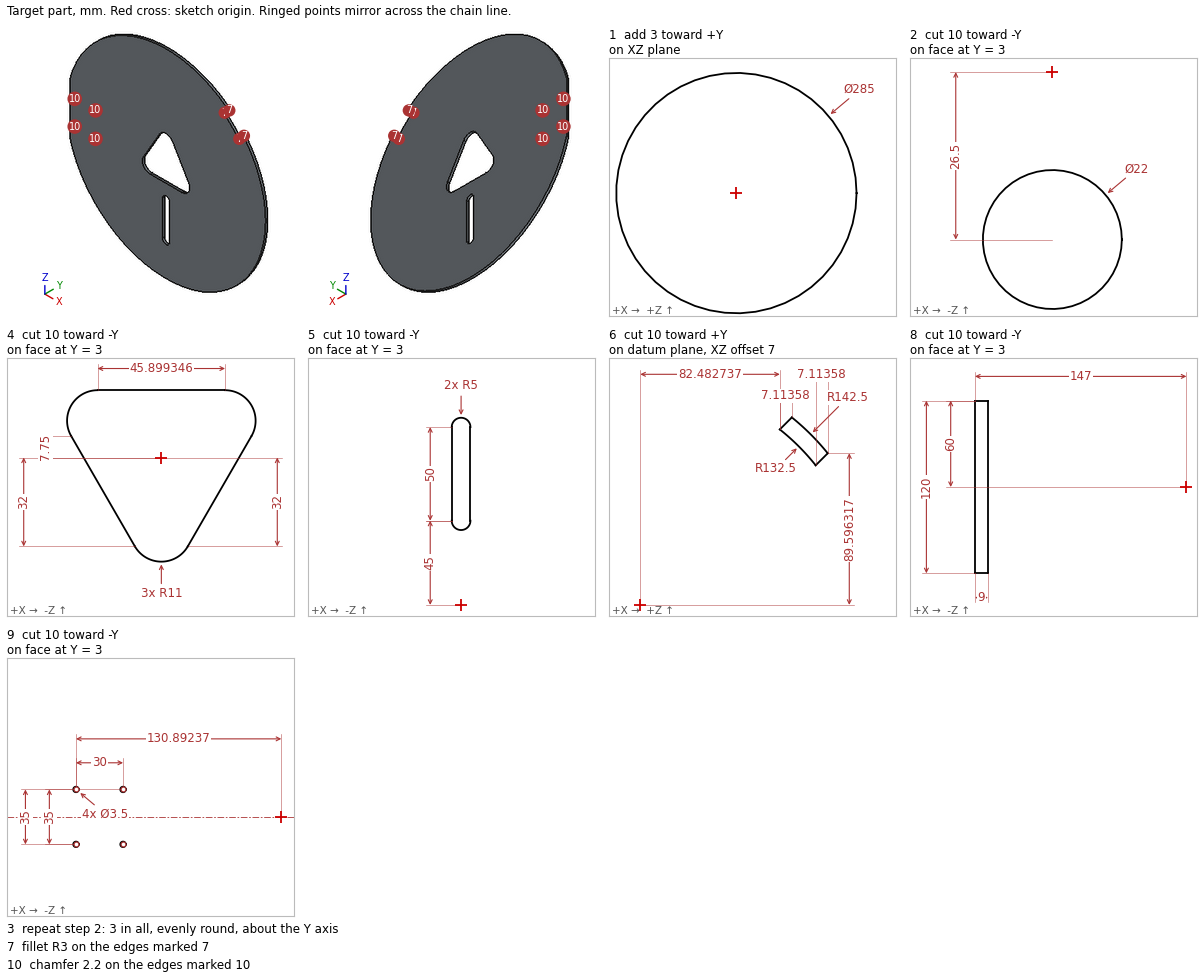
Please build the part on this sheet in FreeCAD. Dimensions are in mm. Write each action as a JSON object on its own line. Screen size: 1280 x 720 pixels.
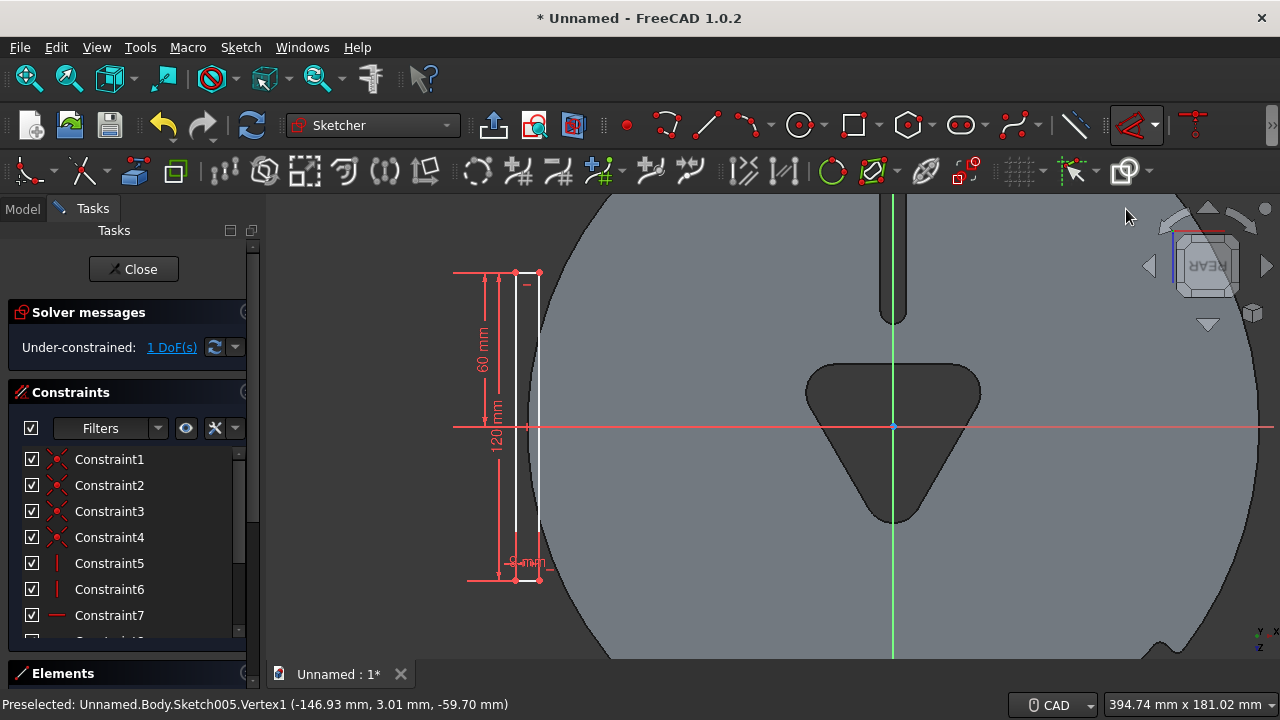
{"action": "left_click", "coordinate": [516, 273]}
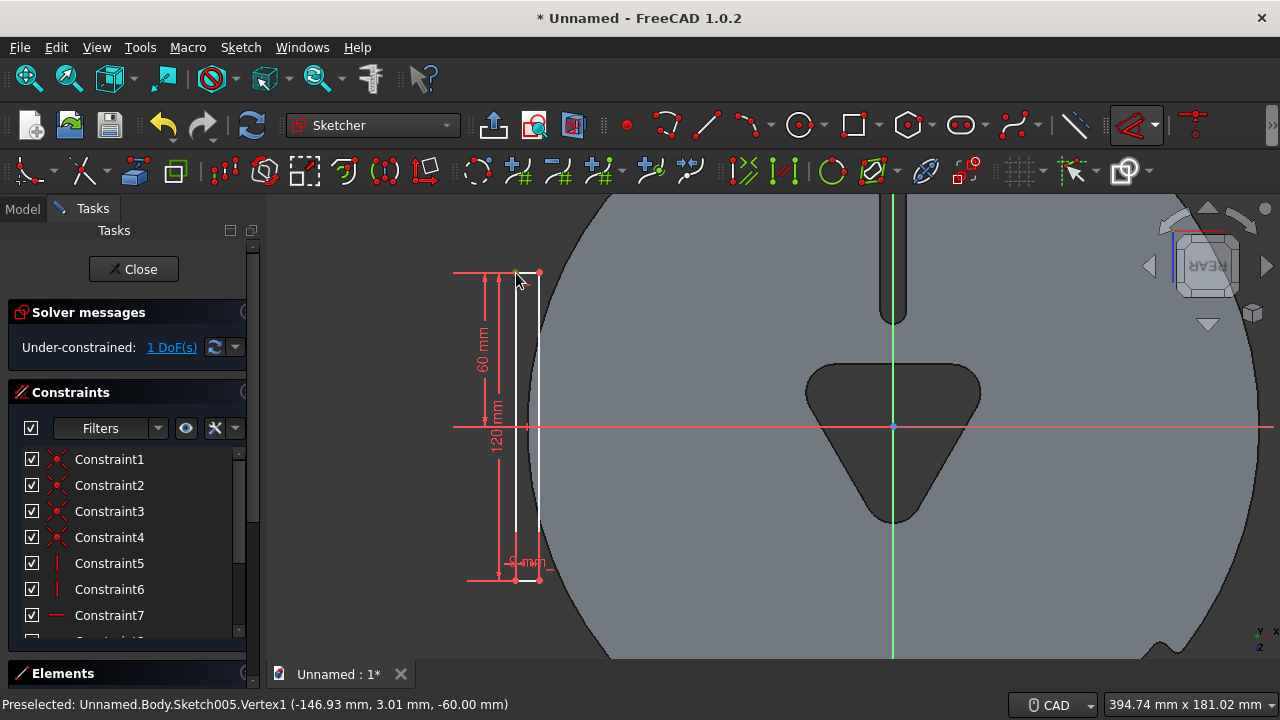
{"action": "left_click", "coordinate": [1158, 126]}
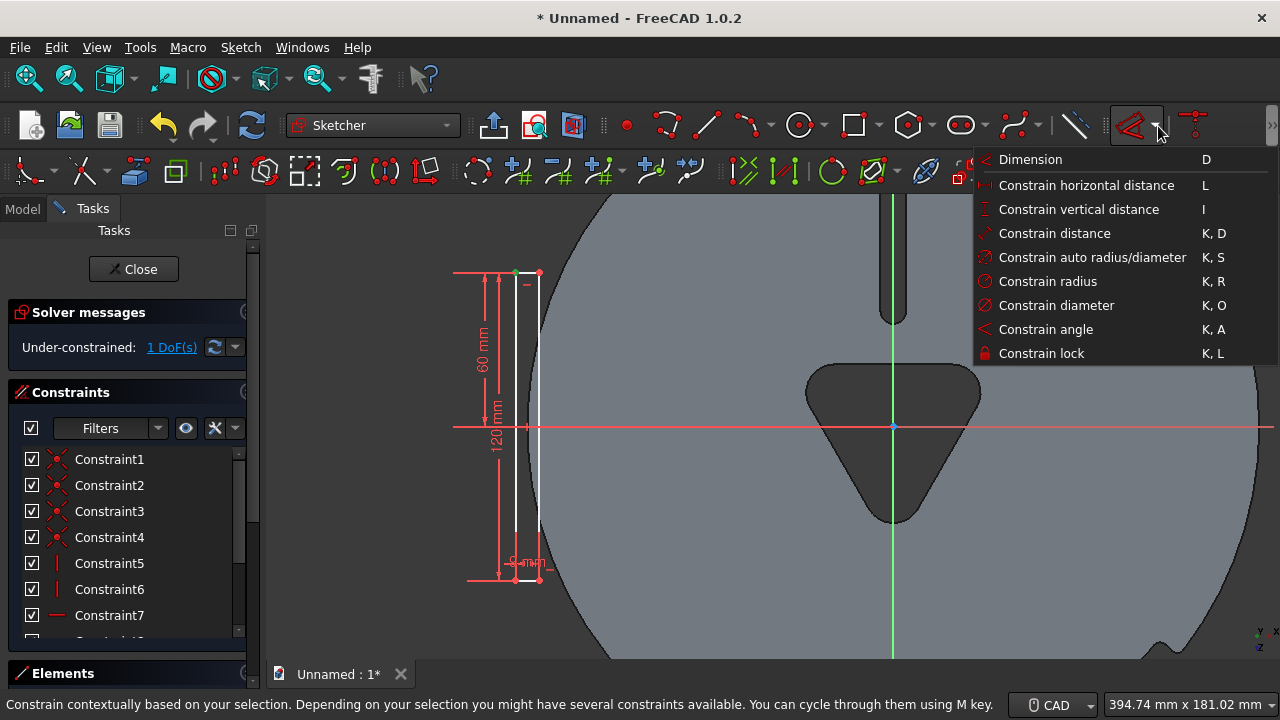
{"action": "left_click", "coordinate": [1126, 185]}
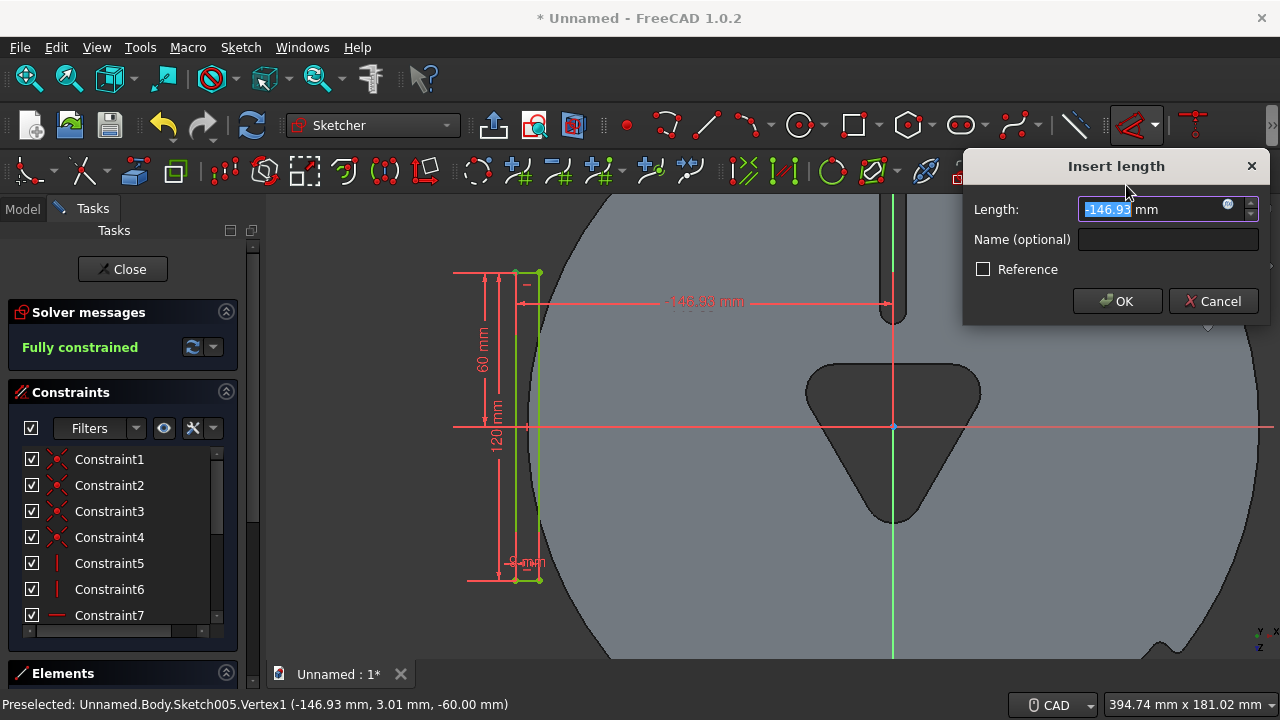
{"action": "type", "text": "-147"}
{"action": "key", "text": "Return"}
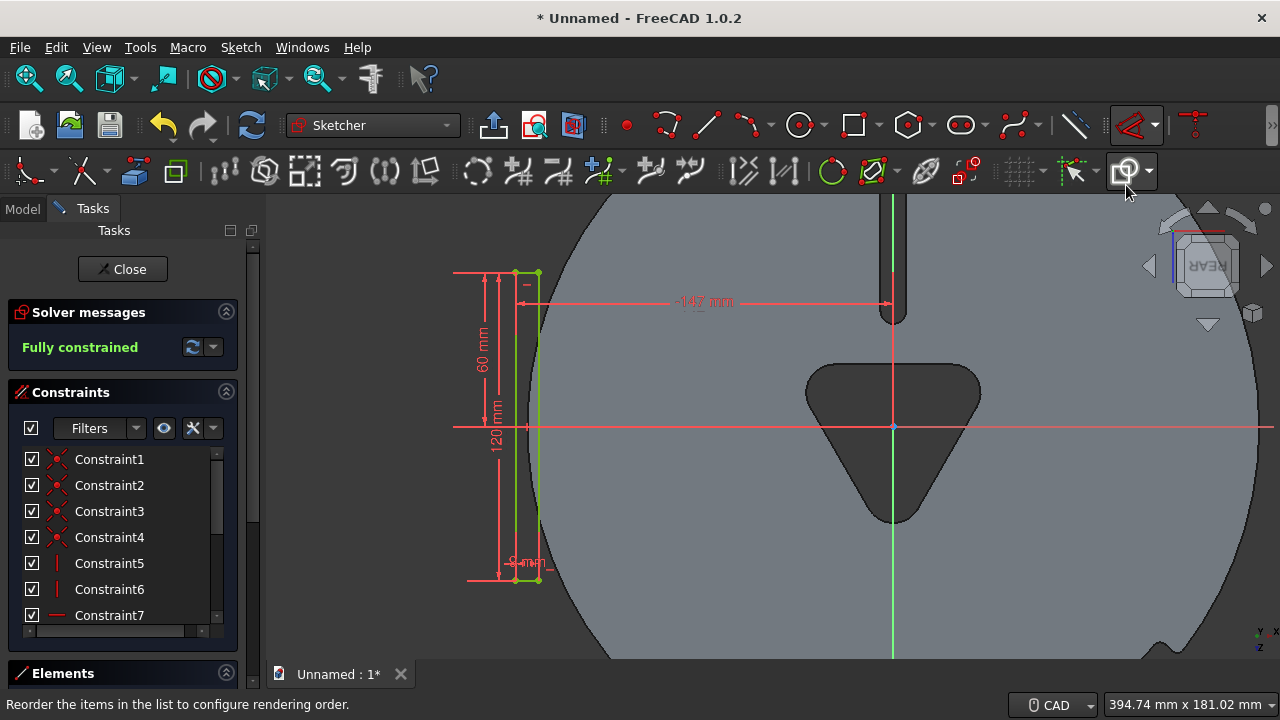
{"action": "left_click", "coordinate": [123, 269]}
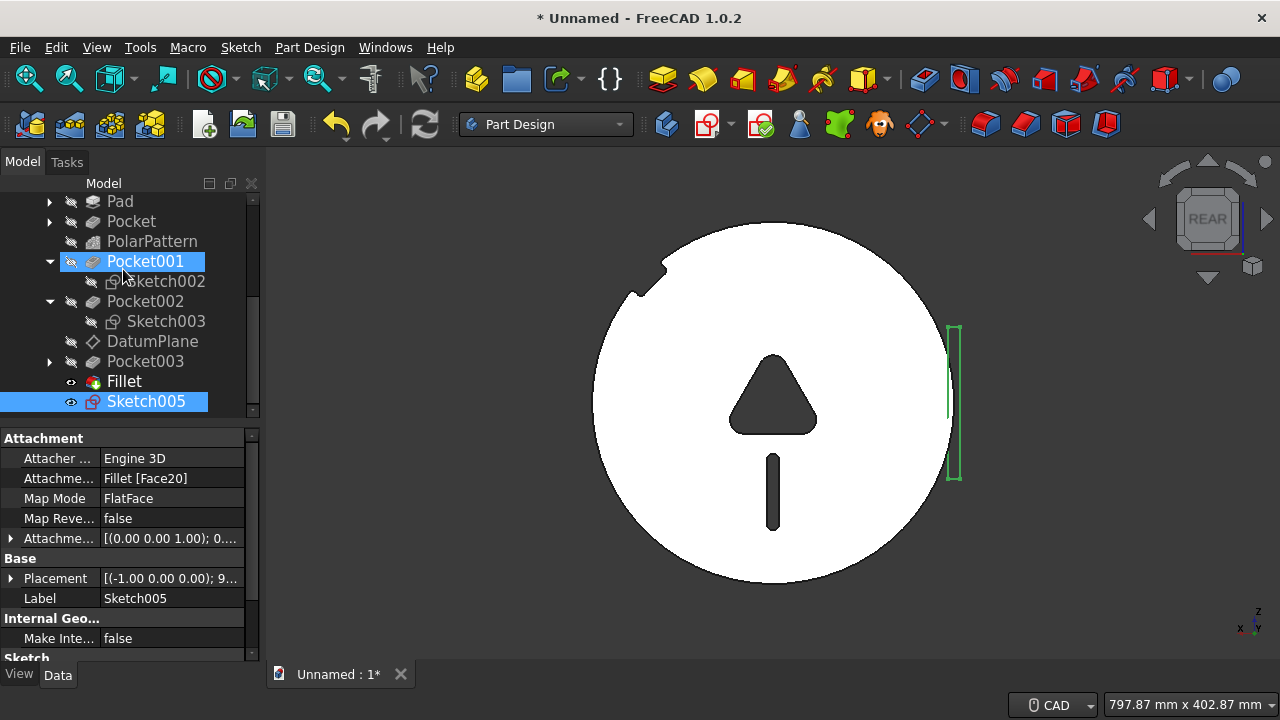
{"action": "left_click", "coordinate": [926, 80]}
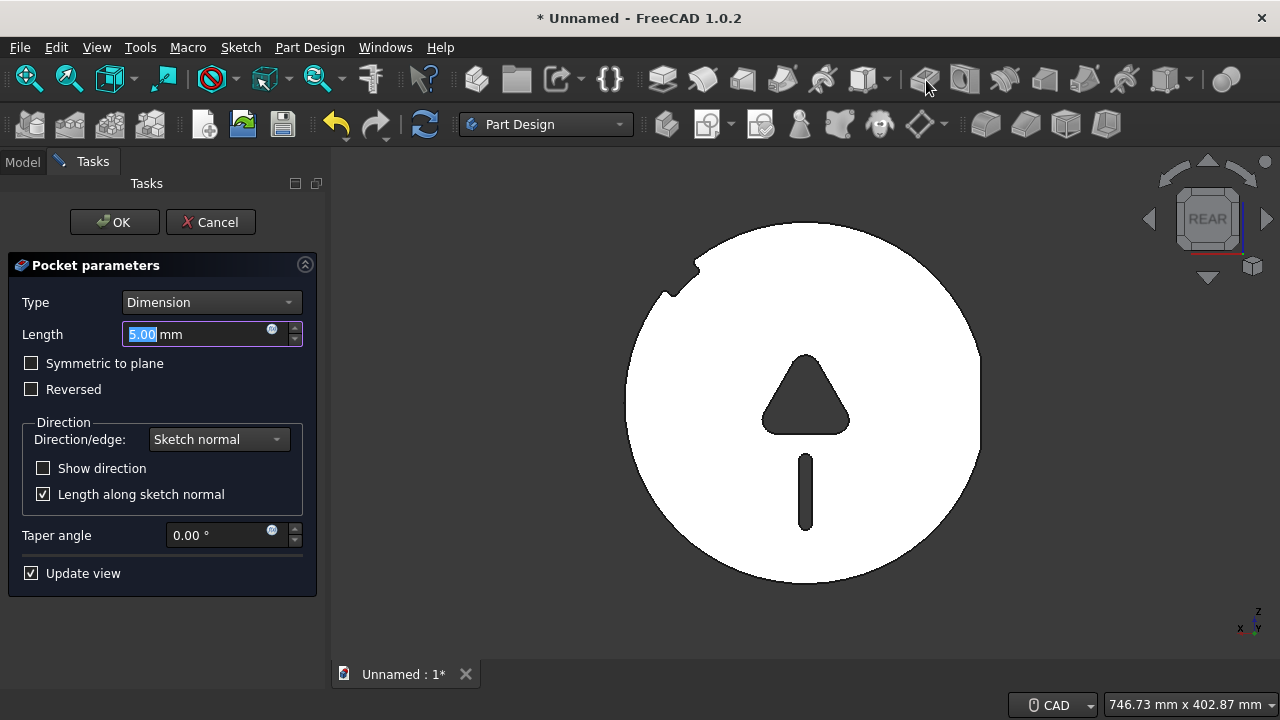
{"action": "type", "text": "10"}
{"action": "key", "text": "Tab"}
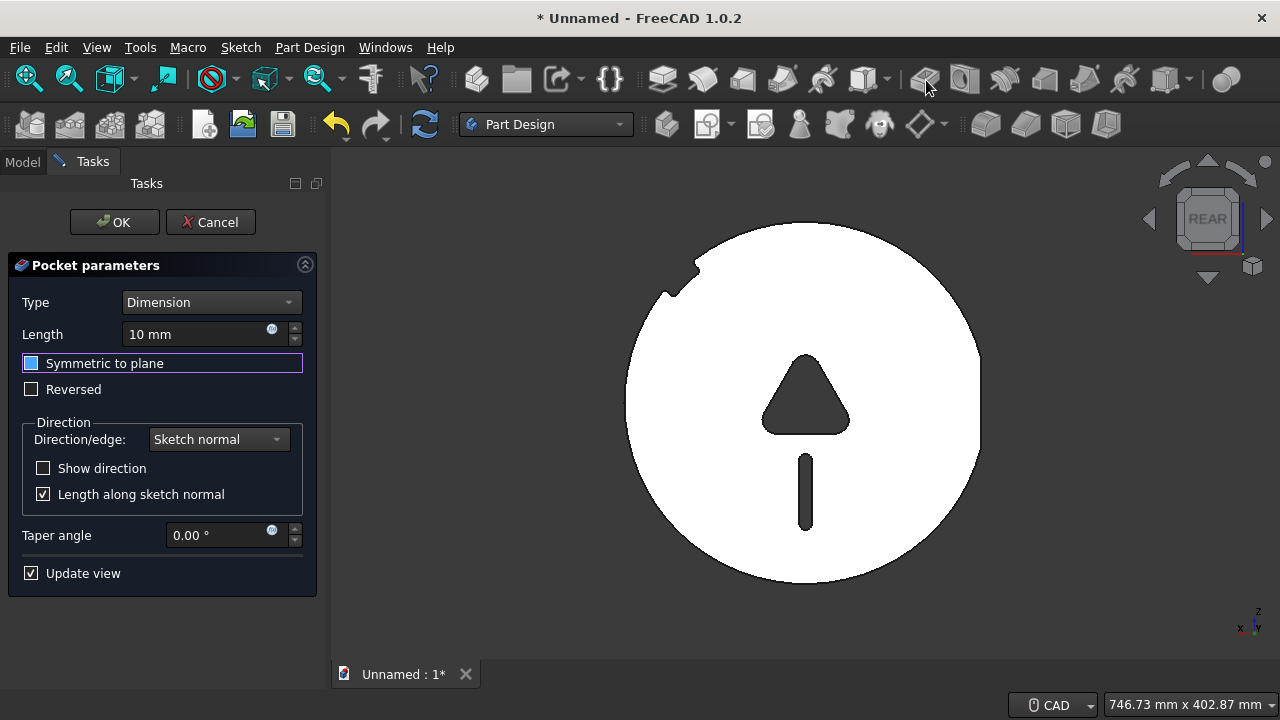
{"action": "left_click", "coordinate": [115, 222]}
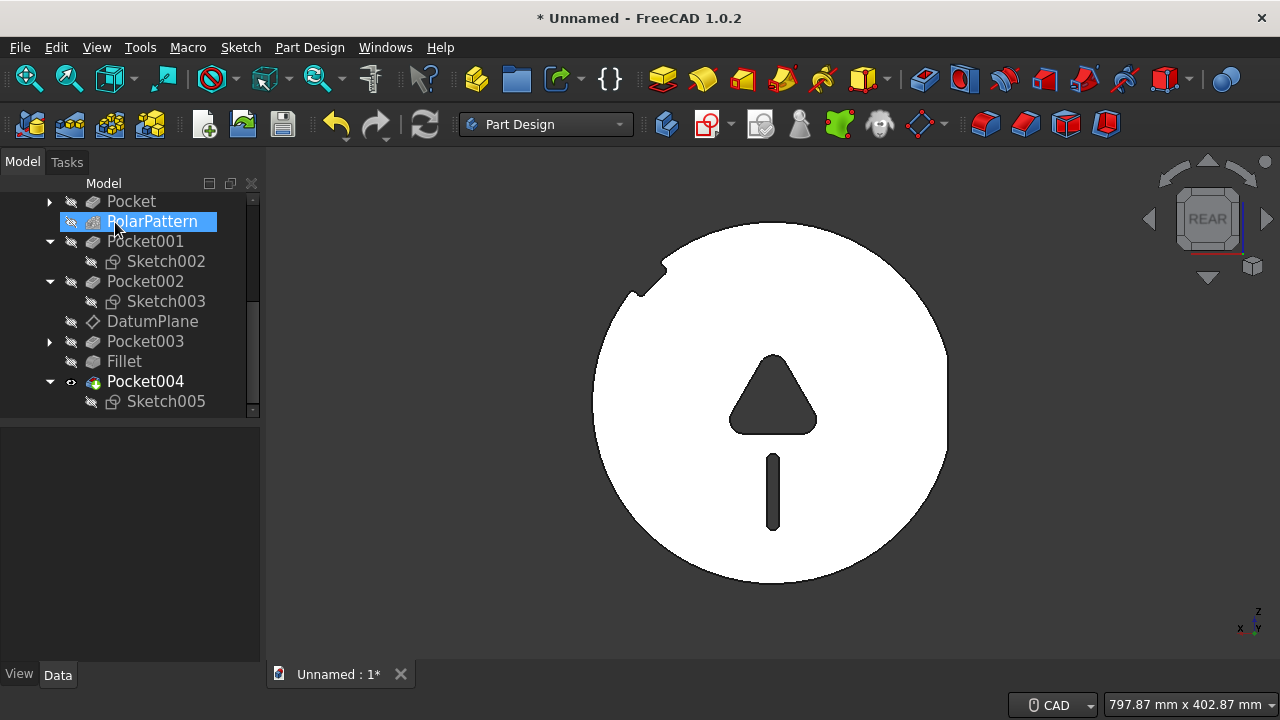
{"action": "left_click", "coordinate": [872, 350]}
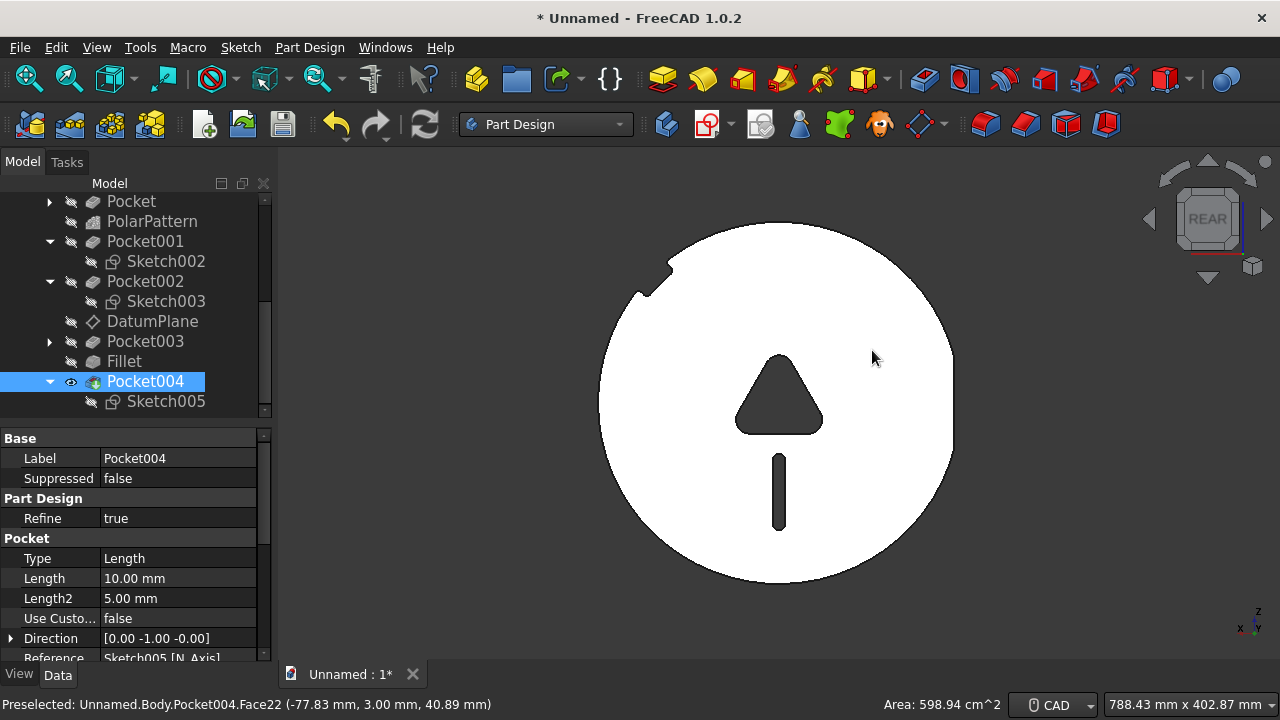
{"action": "left_click", "coordinate": [708, 124]}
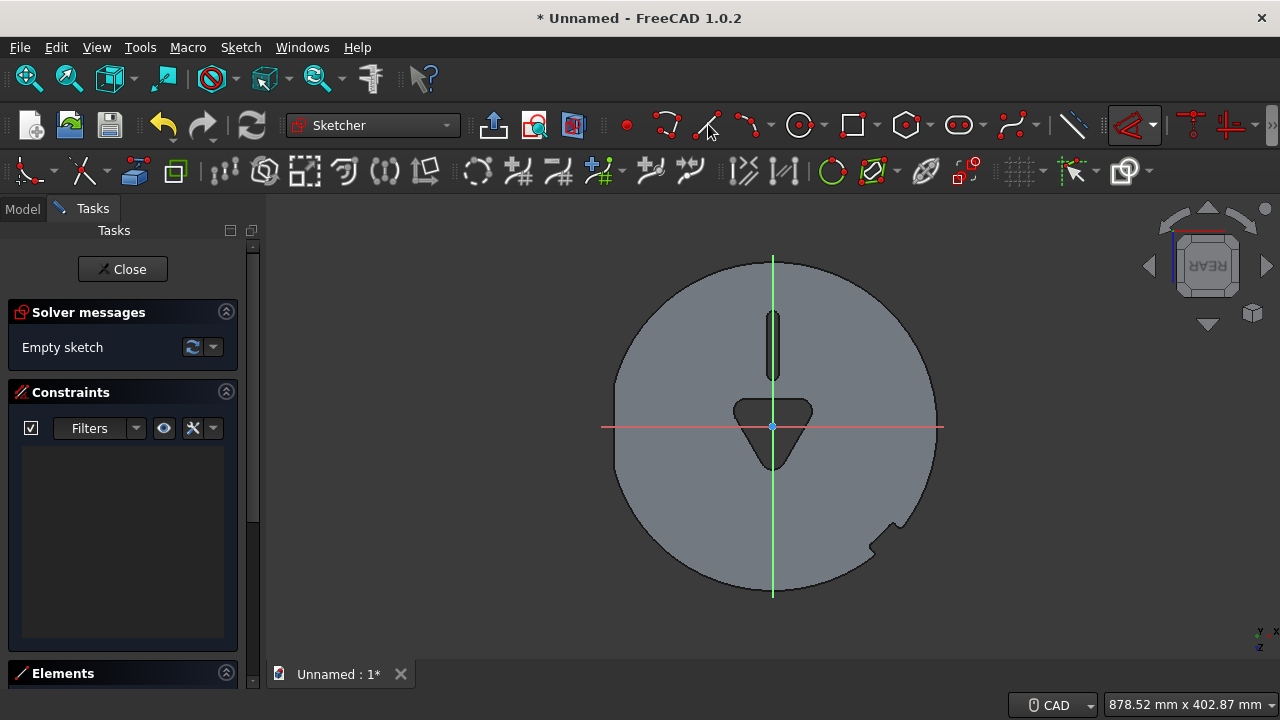
{"action": "scroll", "coordinate": [626, 427], "scroll_direction": "up", "scroll_amount": 9}